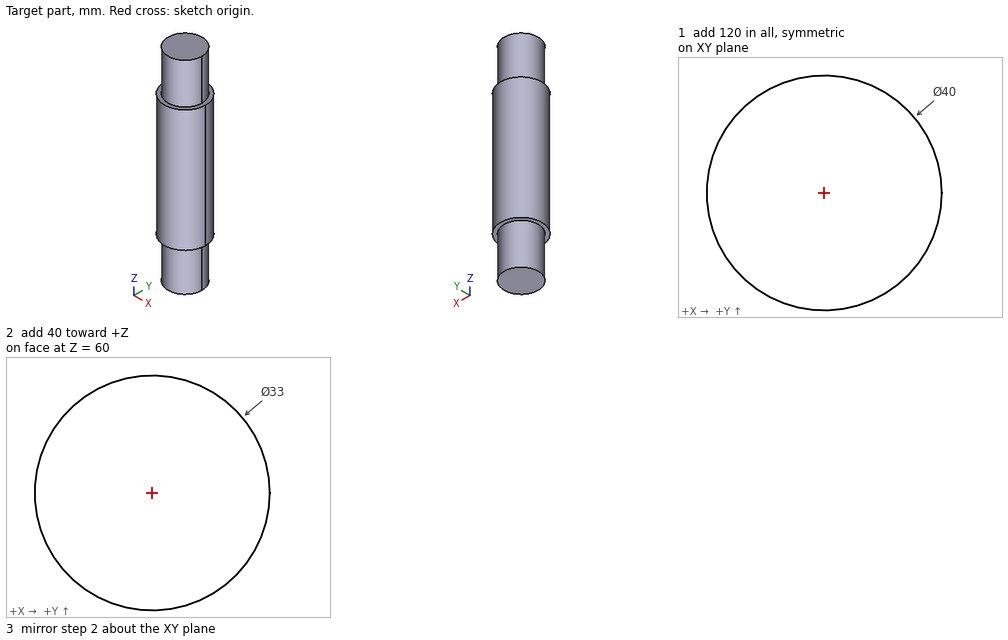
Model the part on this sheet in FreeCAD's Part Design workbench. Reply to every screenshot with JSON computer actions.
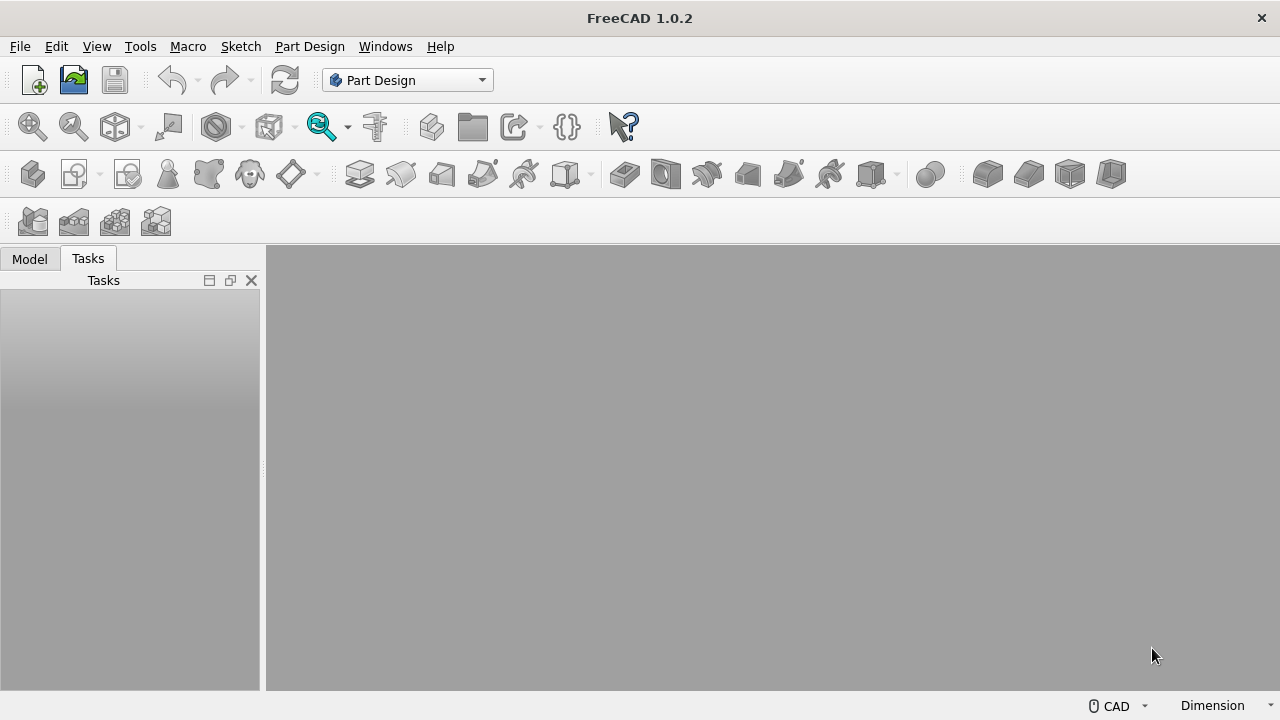
{"action": "left_click", "coordinate": [33, 80]}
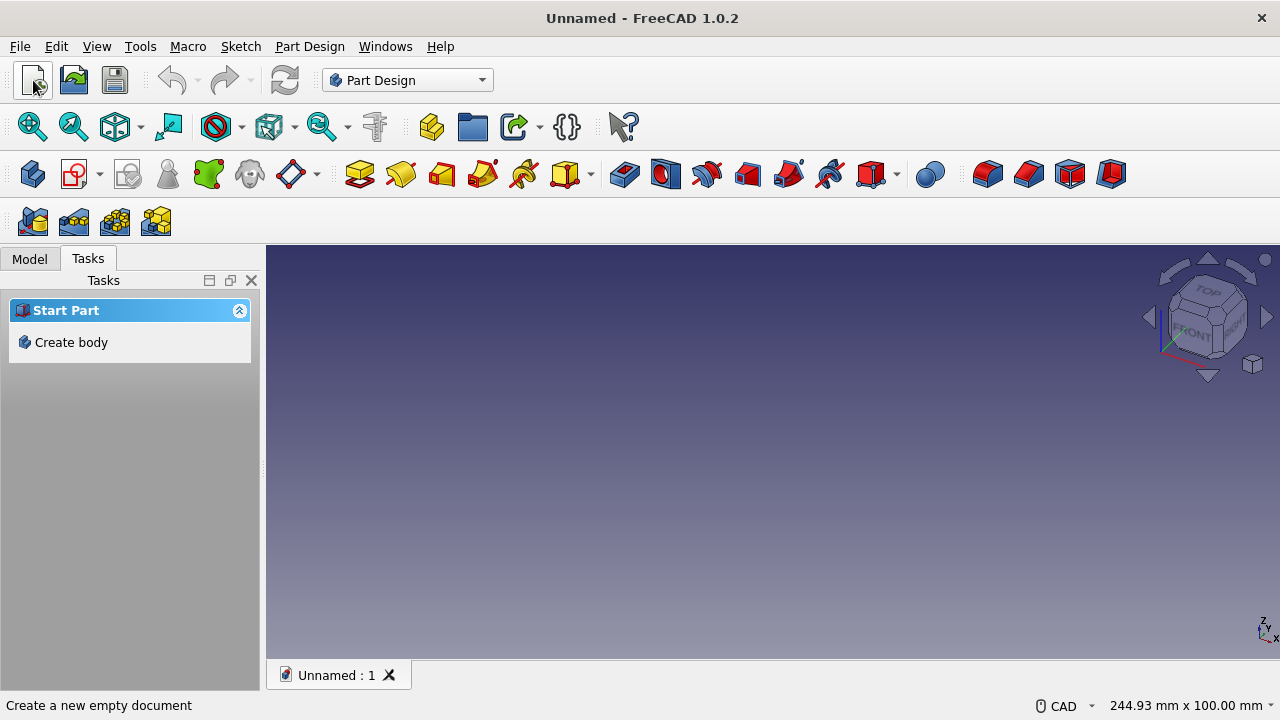
{"action": "left_click", "coordinate": [74, 174]}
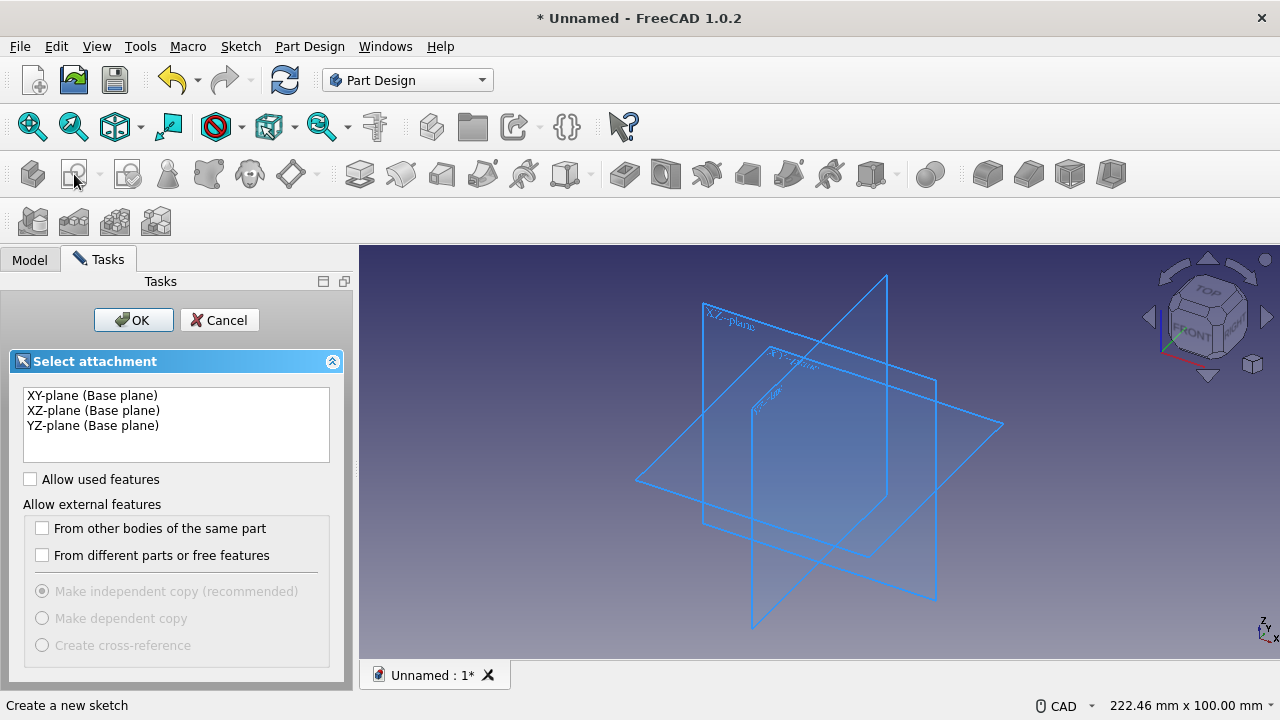
{"action": "left_click", "coordinate": [84, 396]}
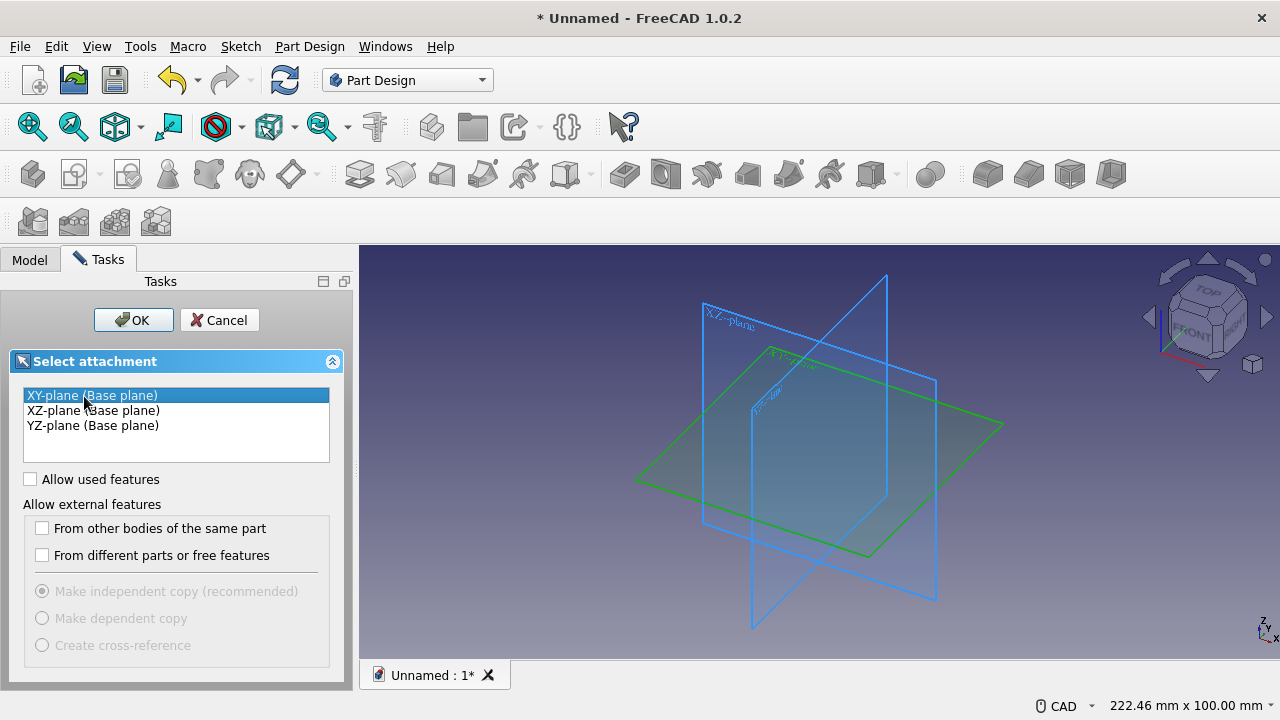
{"action": "left_click", "coordinate": [134, 320]}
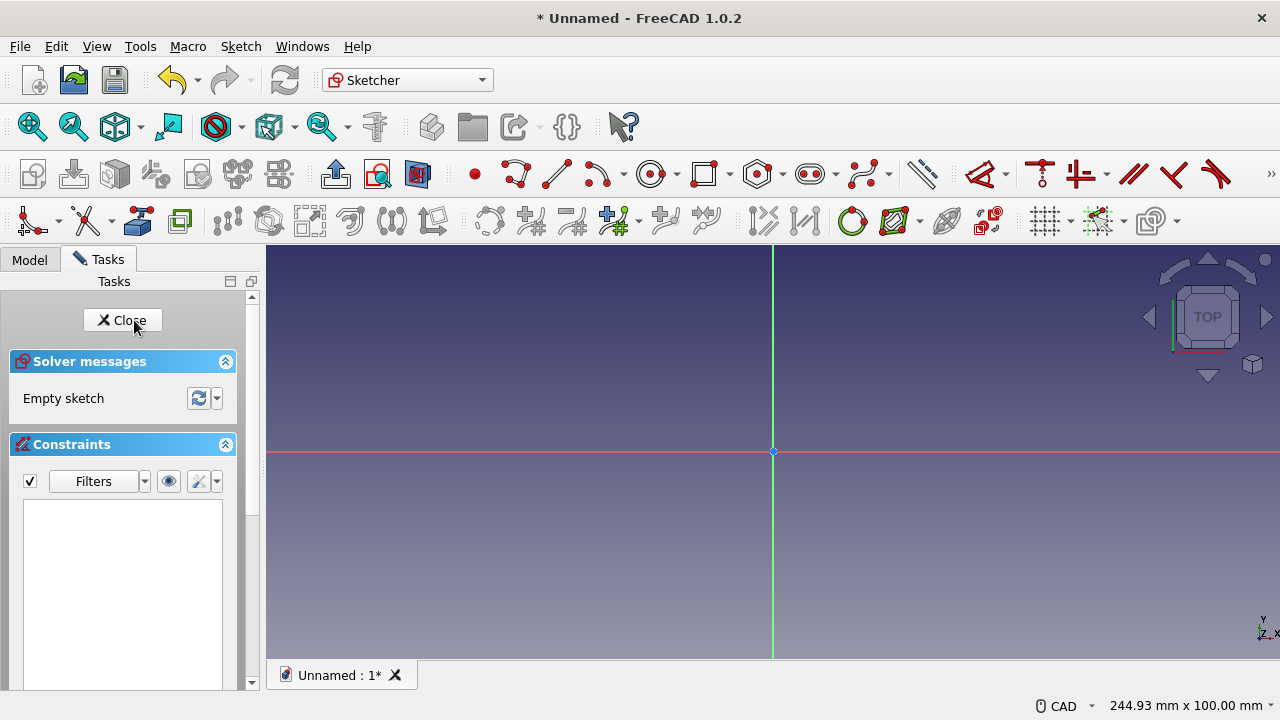
{"action": "scroll", "coordinate": [912, 452], "scroll_direction": "up", "scroll_amount": 2}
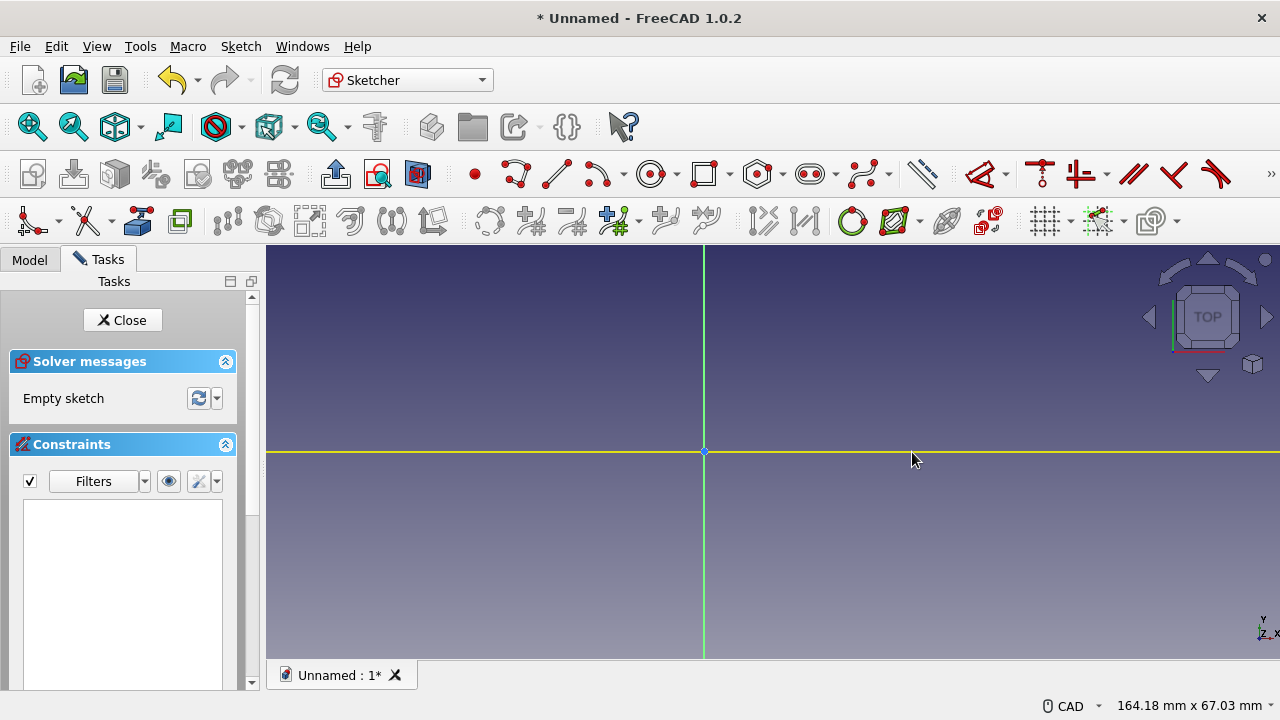
{"action": "left_click", "coordinate": [650, 174]}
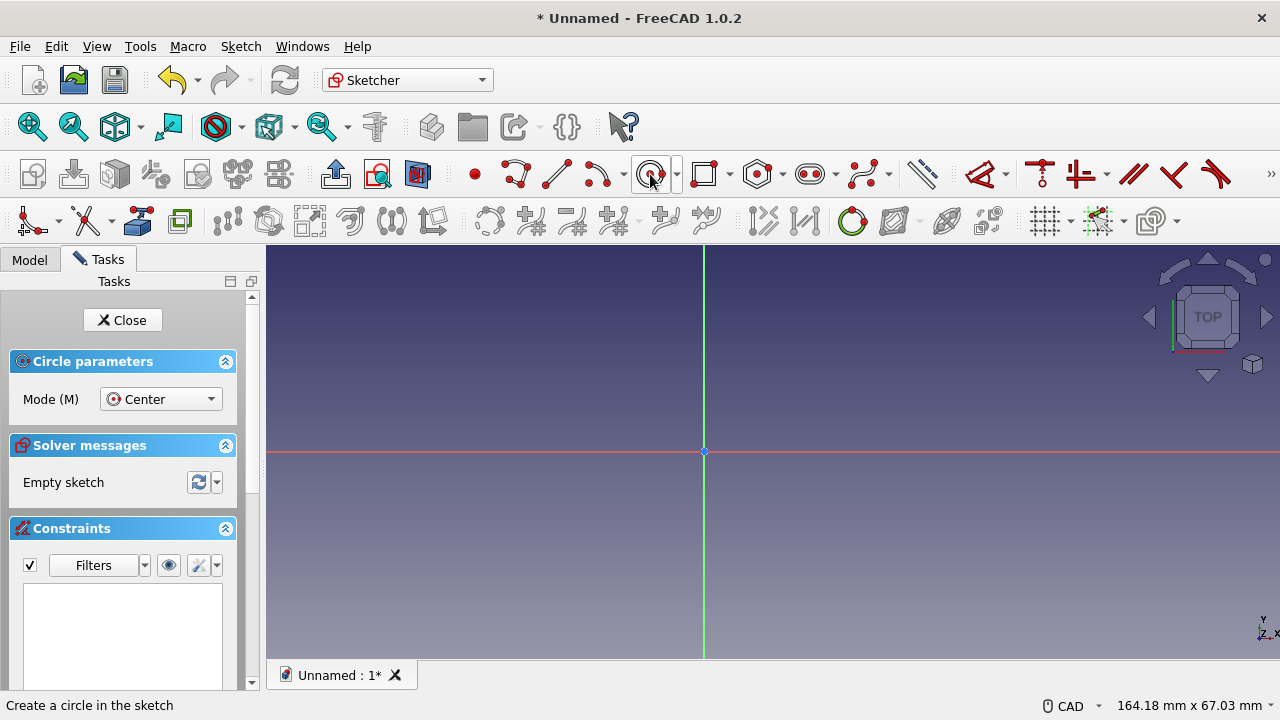
{"action": "left_click", "coordinate": [704, 452]}
{"action": "left_click", "coordinate": [792, 364]}
{"action": "key", "text": "Escape"}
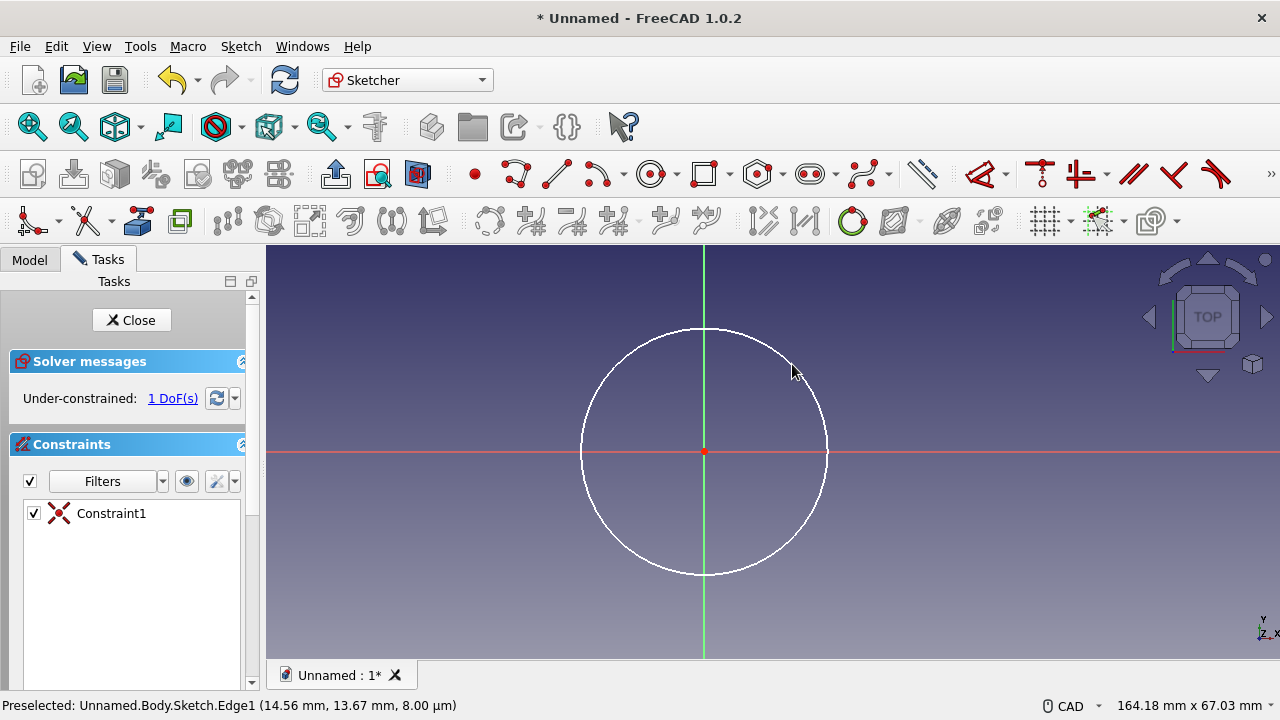
{"action": "left_click", "coordinate": [791, 364]}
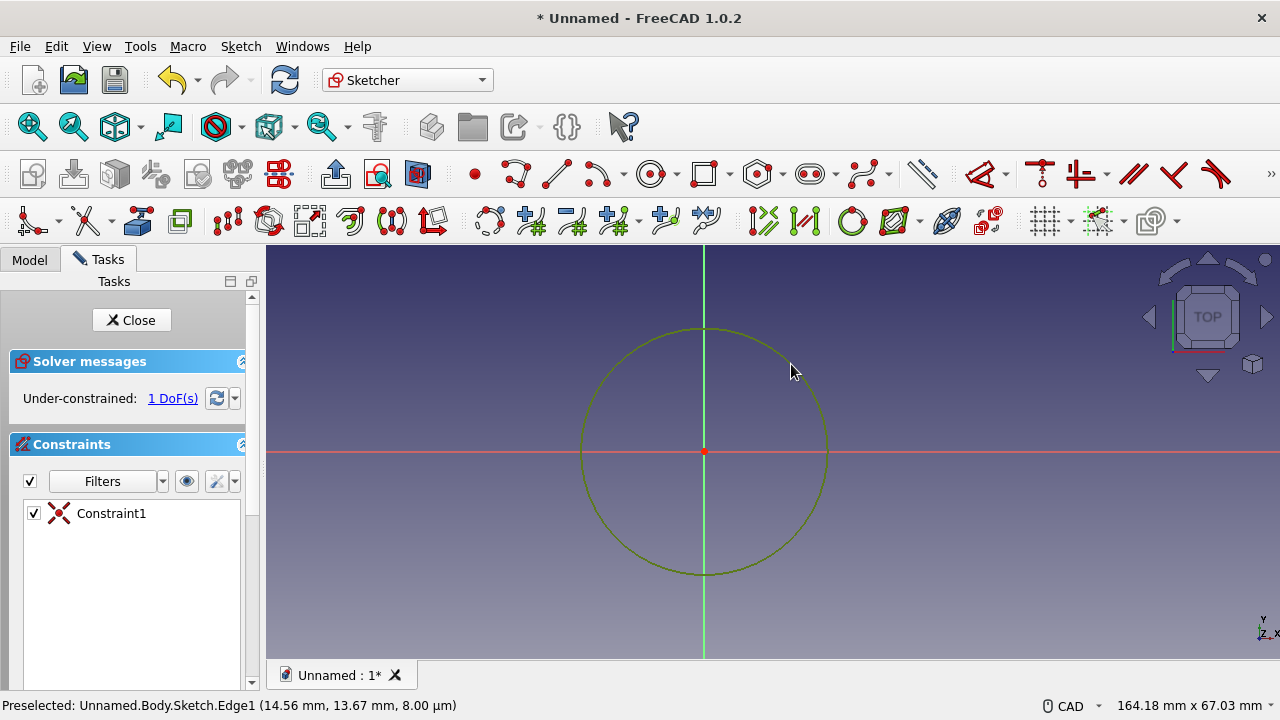
{"action": "key", "text": "k o"}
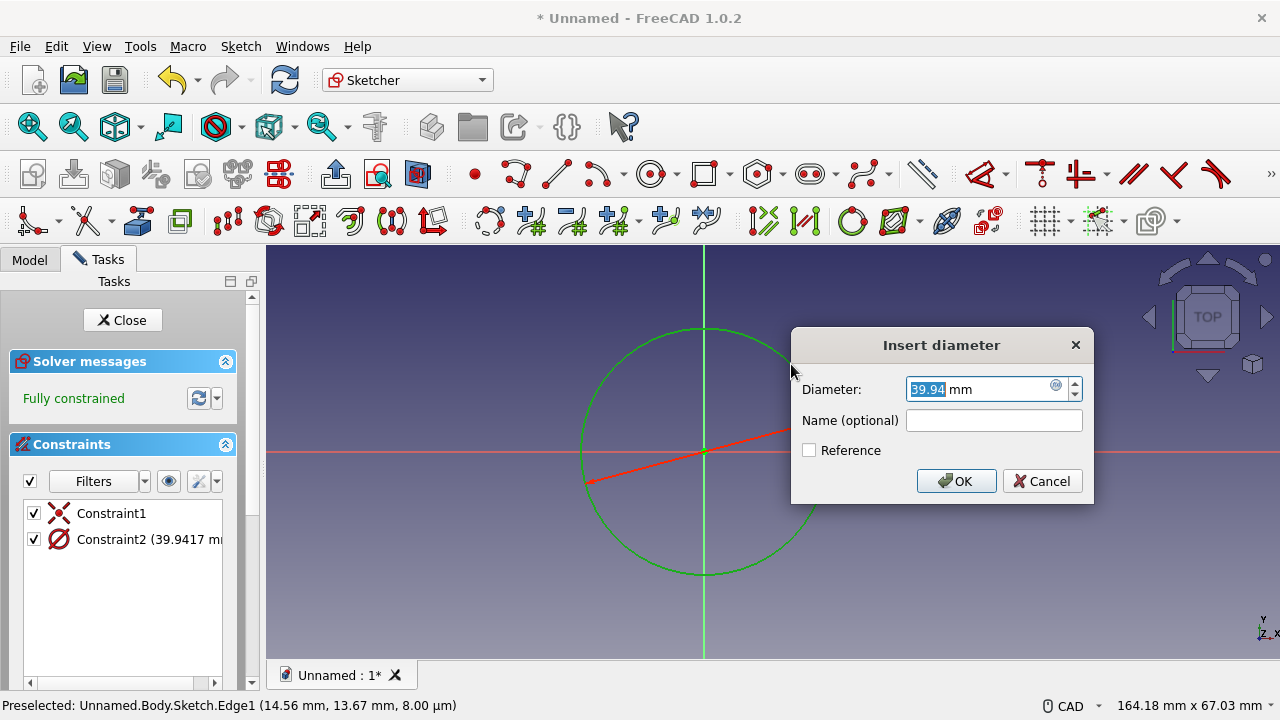
{"action": "type", "text": "40"}
{"action": "key", "text": "Return"}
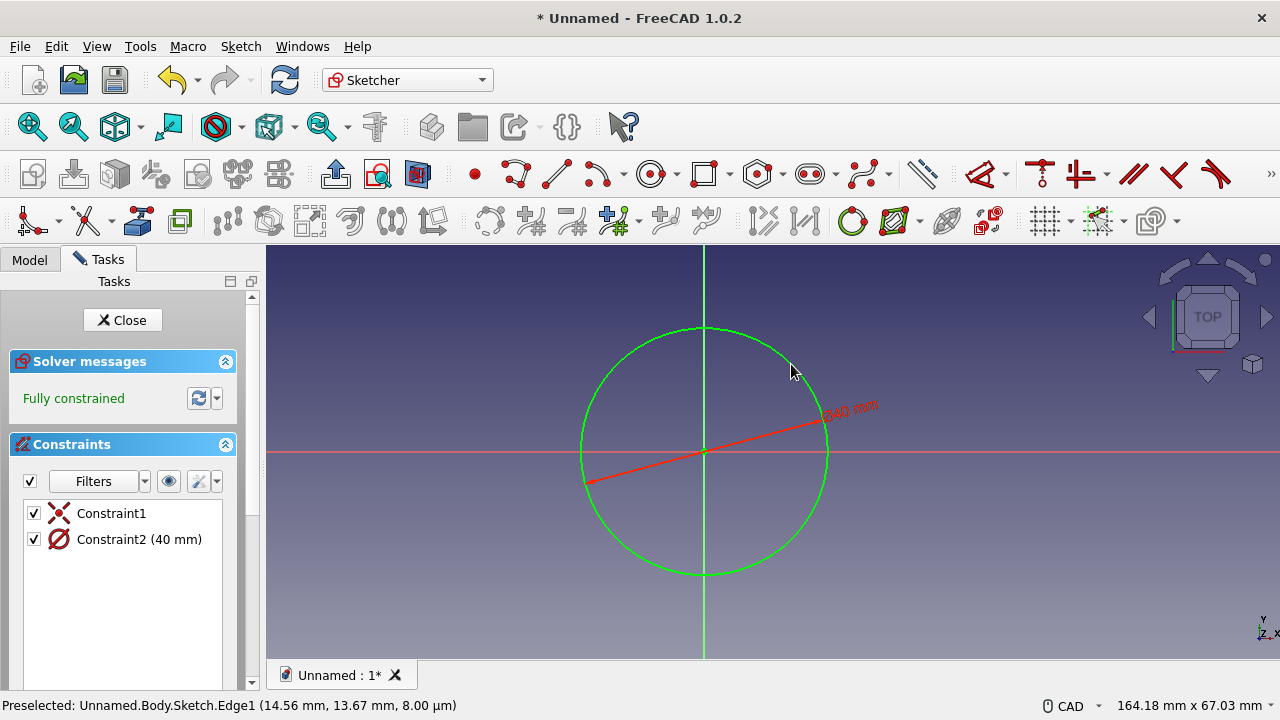
{"action": "left_click", "coordinate": [123, 320]}